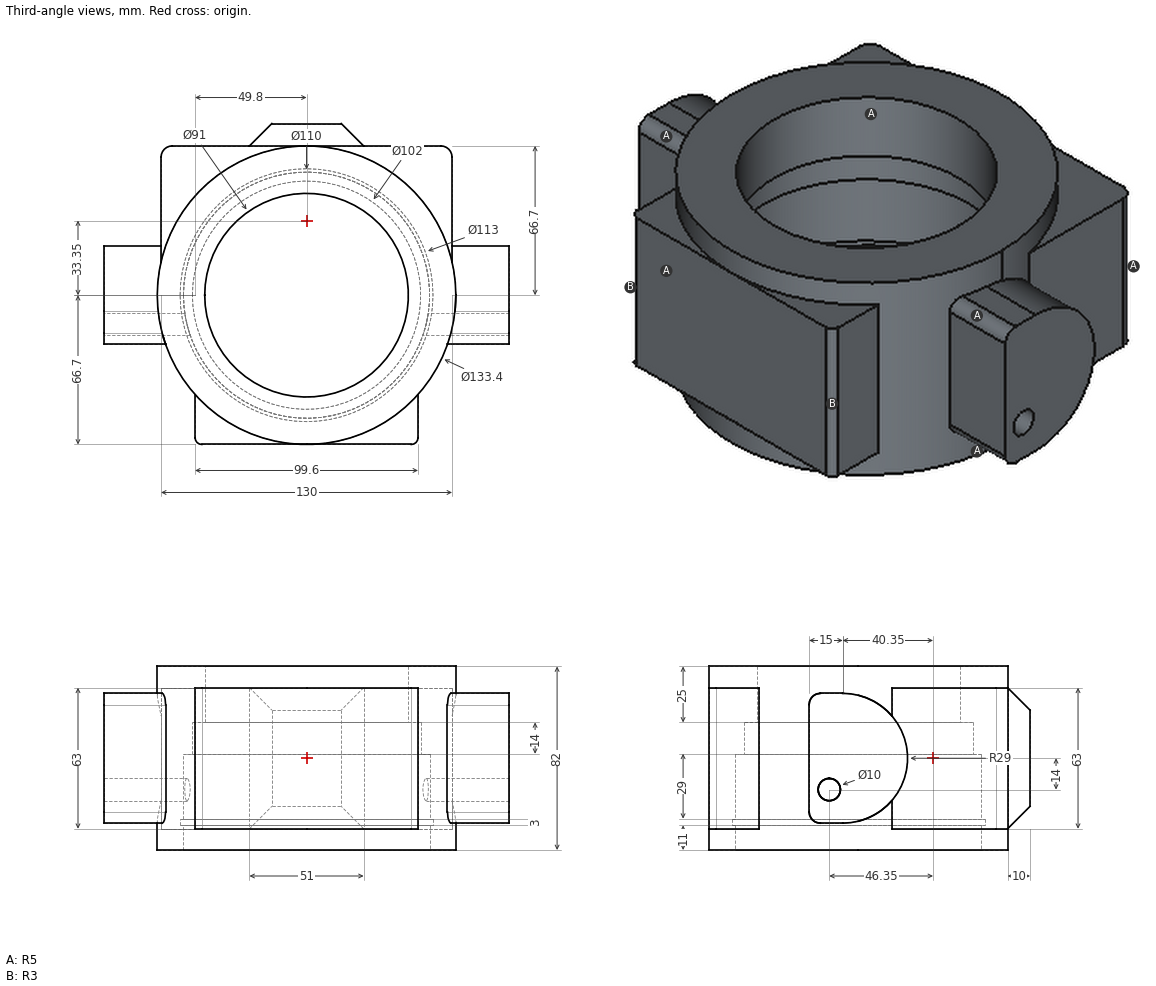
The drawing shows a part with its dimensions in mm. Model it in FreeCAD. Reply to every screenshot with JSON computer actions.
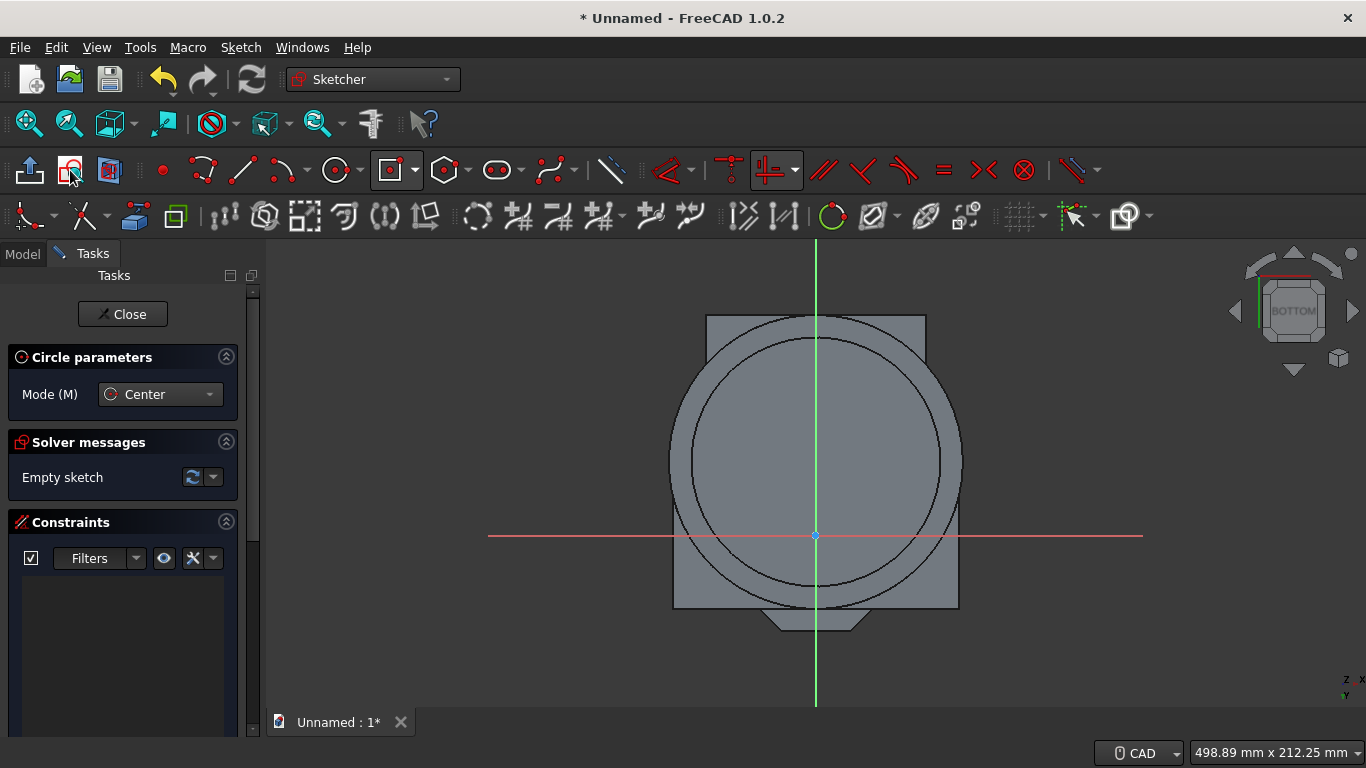
{"action": "left_click", "coordinate": [816, 462]}
{"action": "left_click", "coordinate": [902, 376]}
{"action": "key", "text": "Escape"}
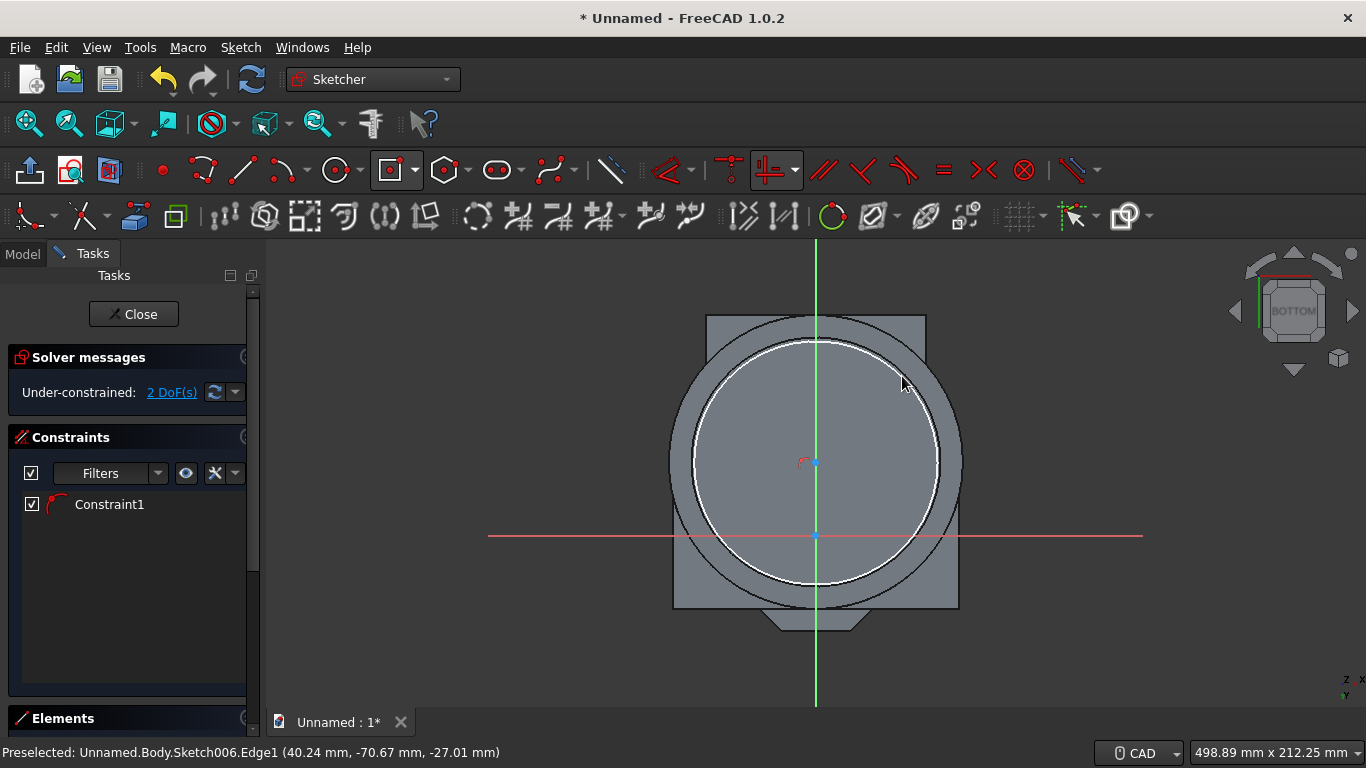
{"action": "key", "text": "d"}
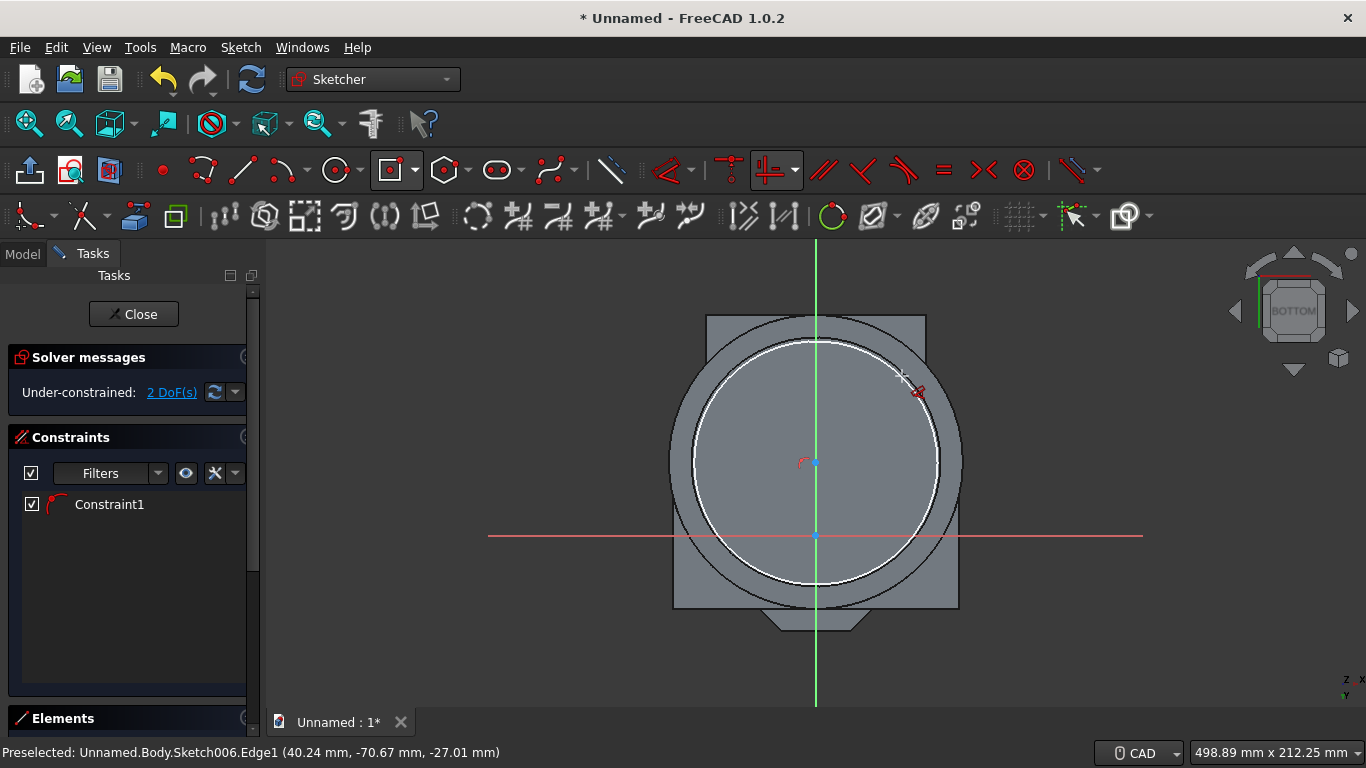
{"action": "left_click", "coordinate": [902, 377]}
{"action": "left_click", "coordinate": [925, 354]}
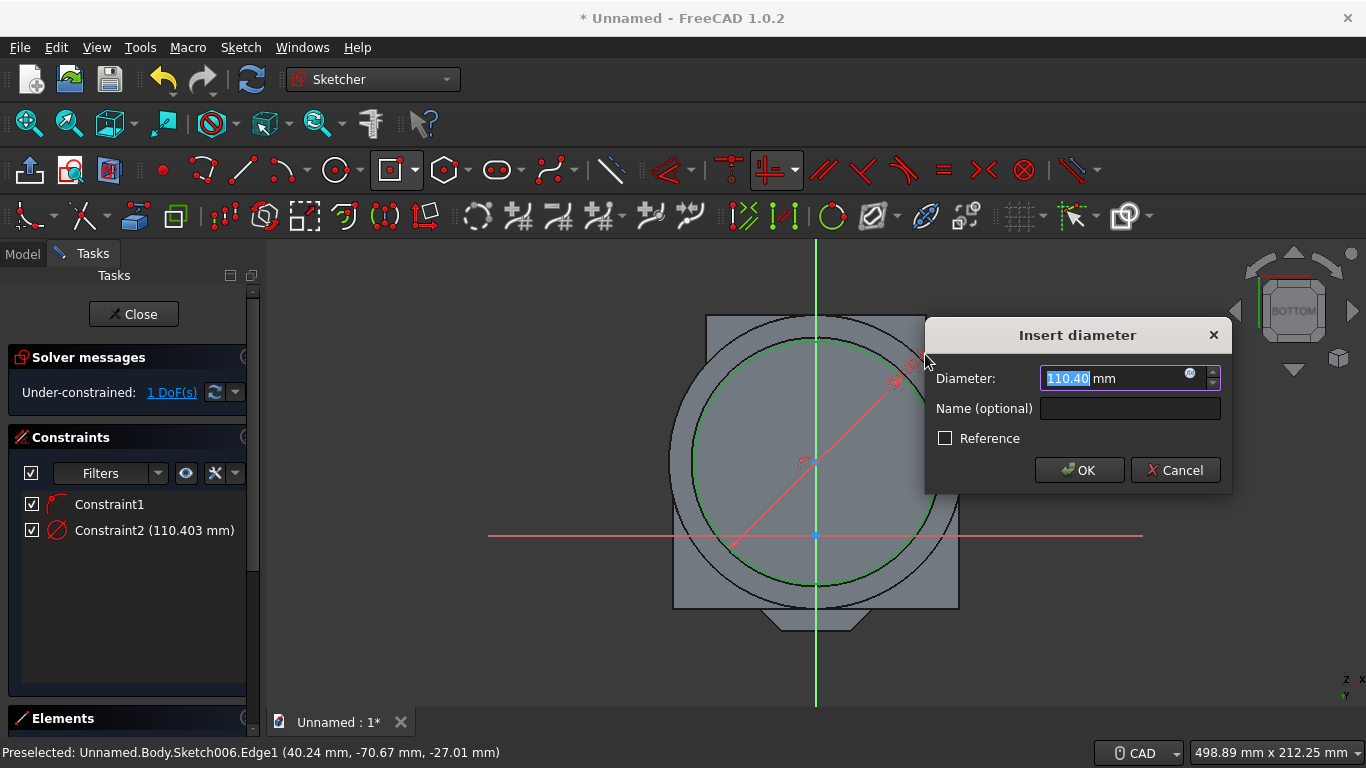
{"action": "type", "text": "110"}
{"action": "key", "text": "Return"}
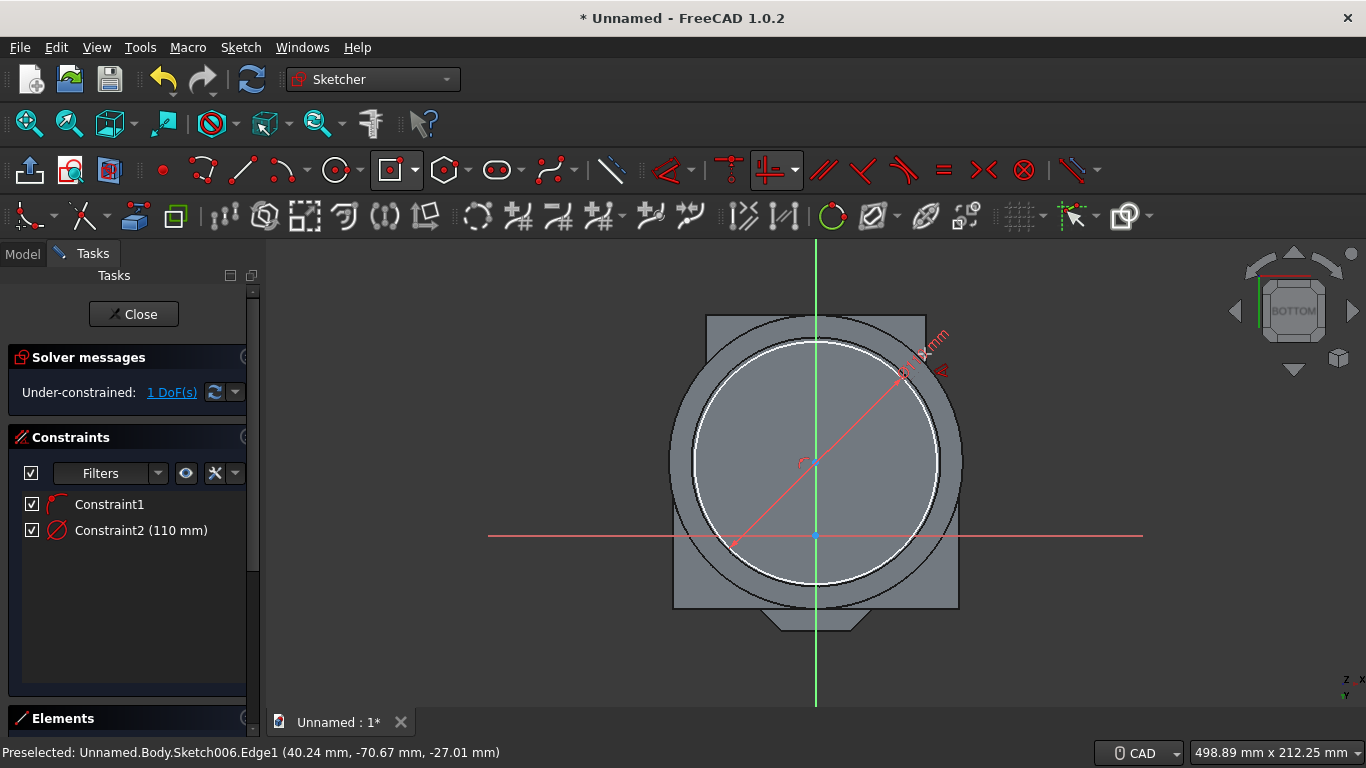
{"action": "left_click", "coordinate": [816, 463]}
{"action": "left_click", "coordinate": [850, 499]}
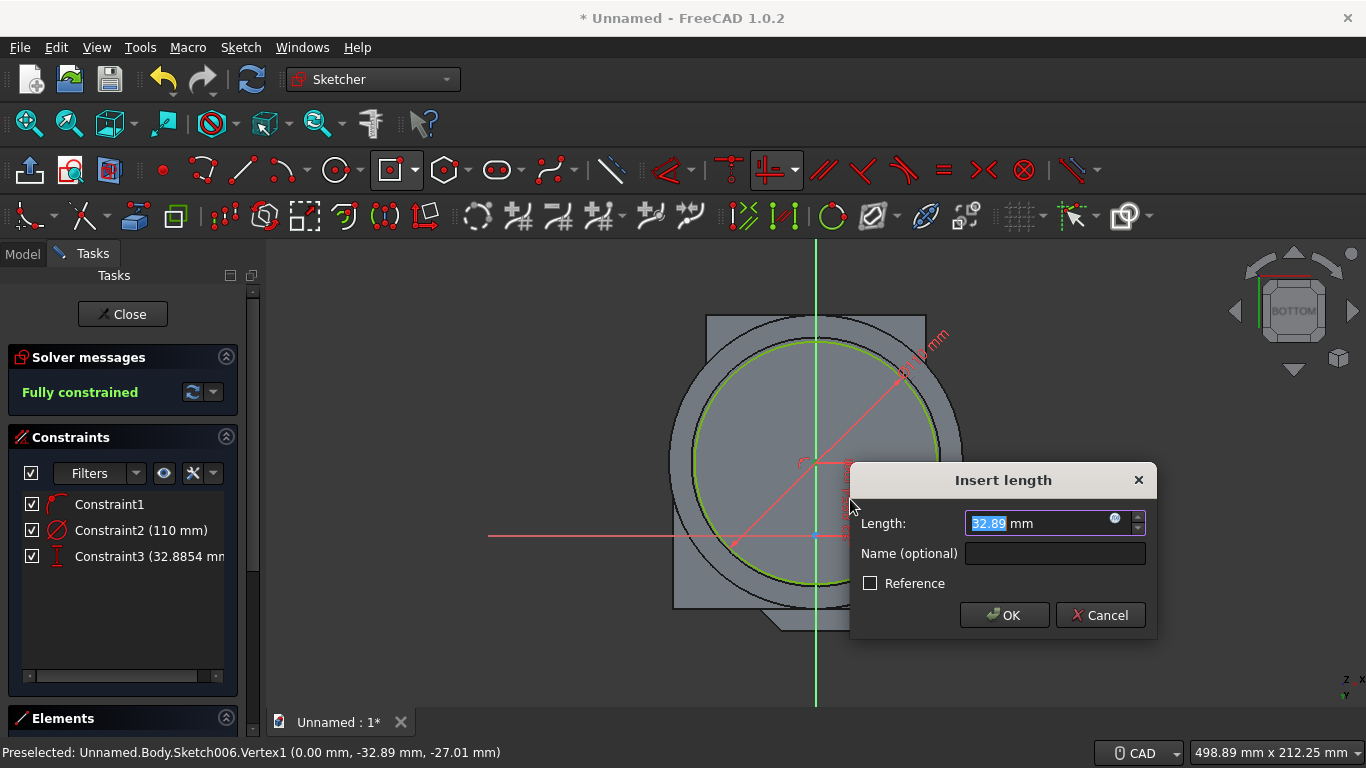
{"action": "type", "text": "33.35"}
{"action": "key", "text": "Return"}
{"action": "key", "text": "Escape"}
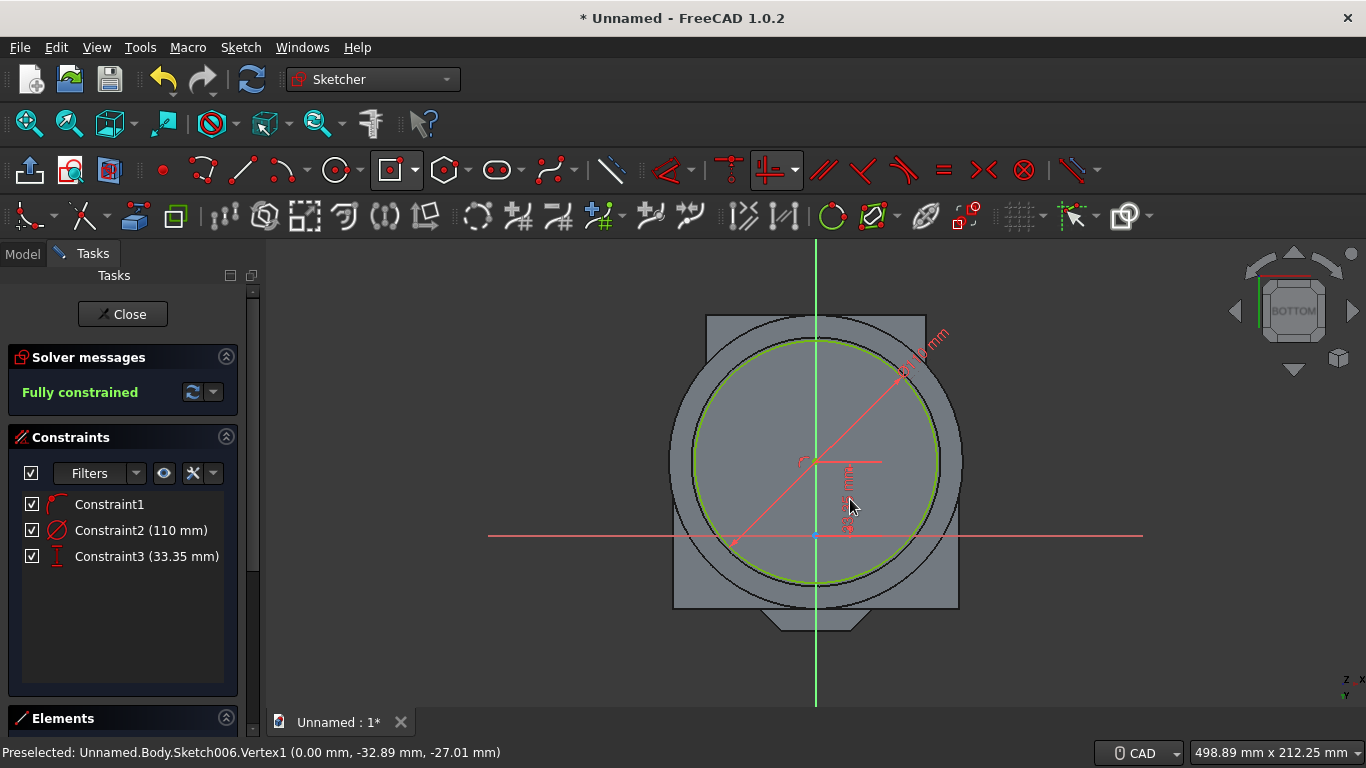
{"action": "left_click", "coordinate": [123, 314]}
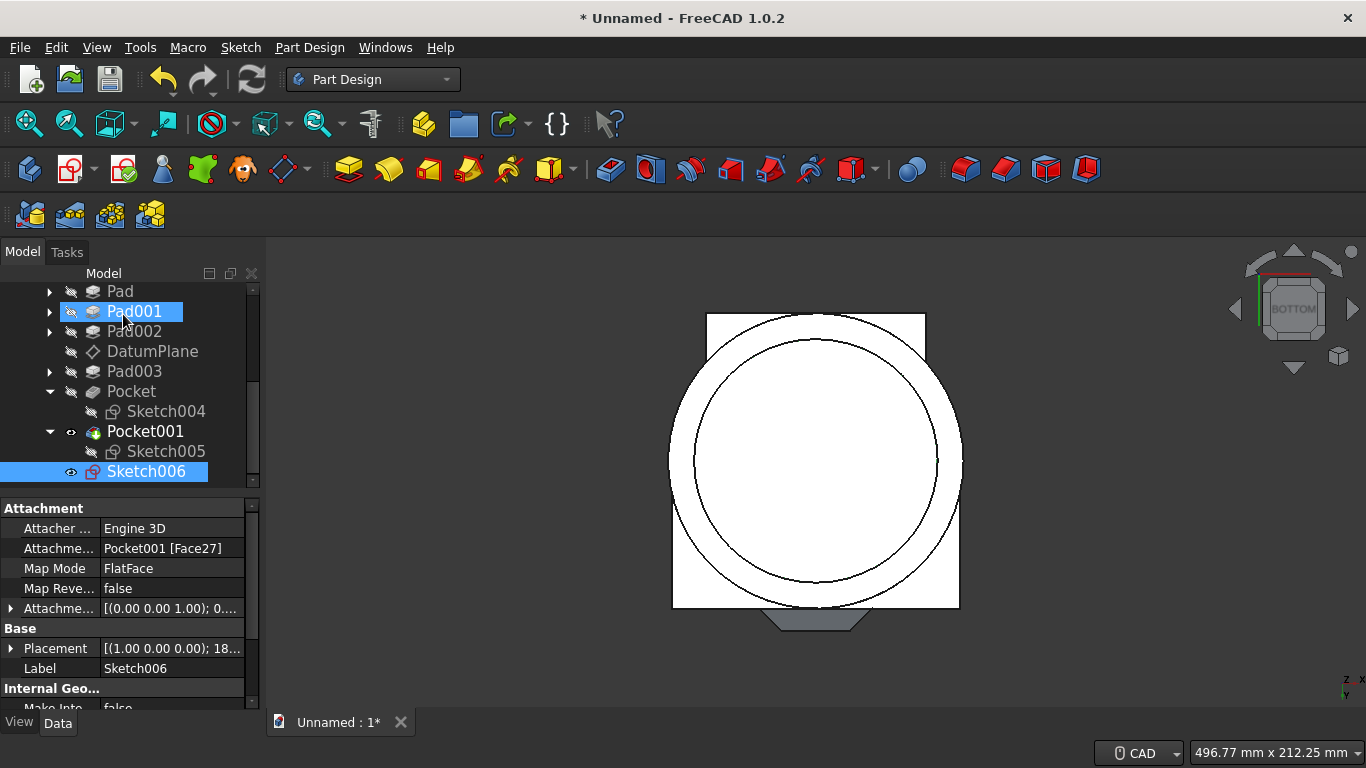
{"action": "left_click", "coordinate": [612, 170]}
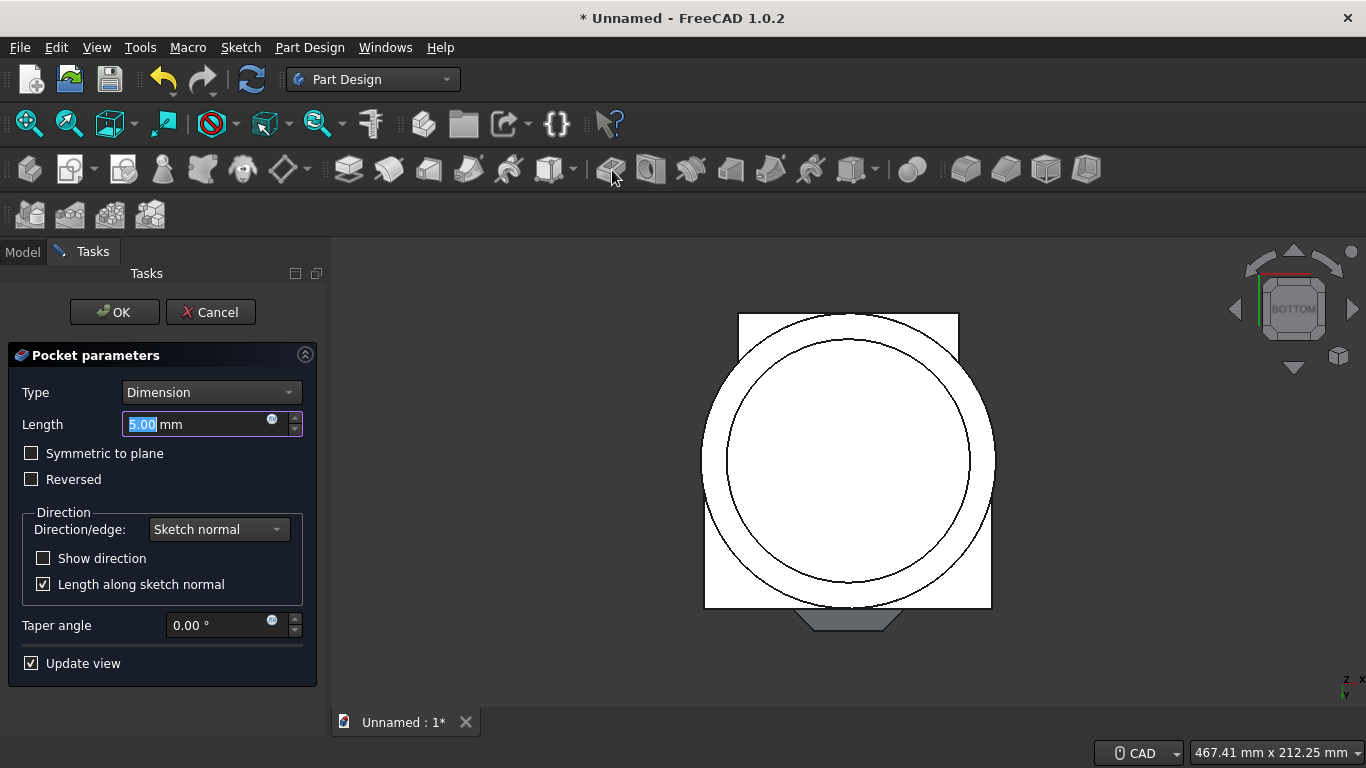
{"action": "type", "text": "29"}
{"action": "key", "text": "Tab"}